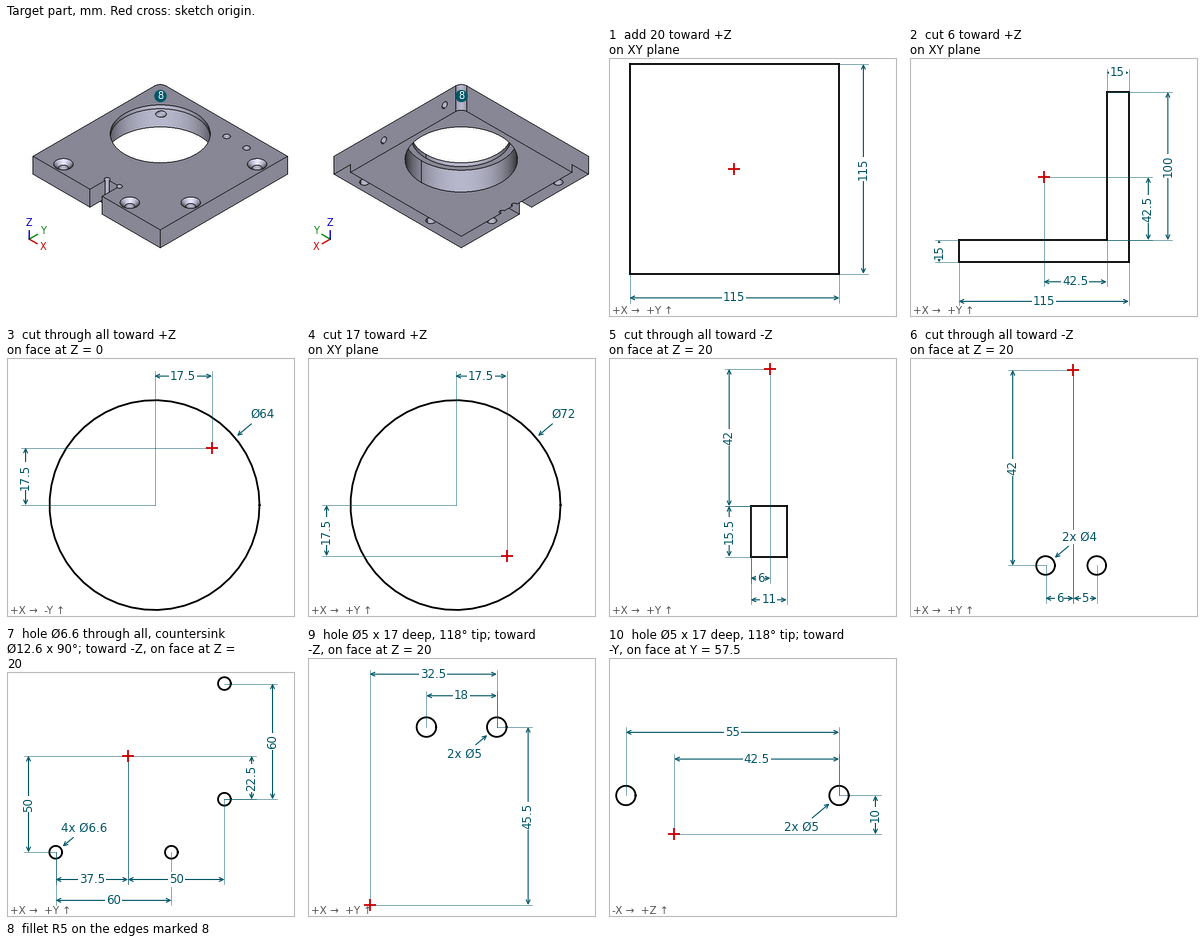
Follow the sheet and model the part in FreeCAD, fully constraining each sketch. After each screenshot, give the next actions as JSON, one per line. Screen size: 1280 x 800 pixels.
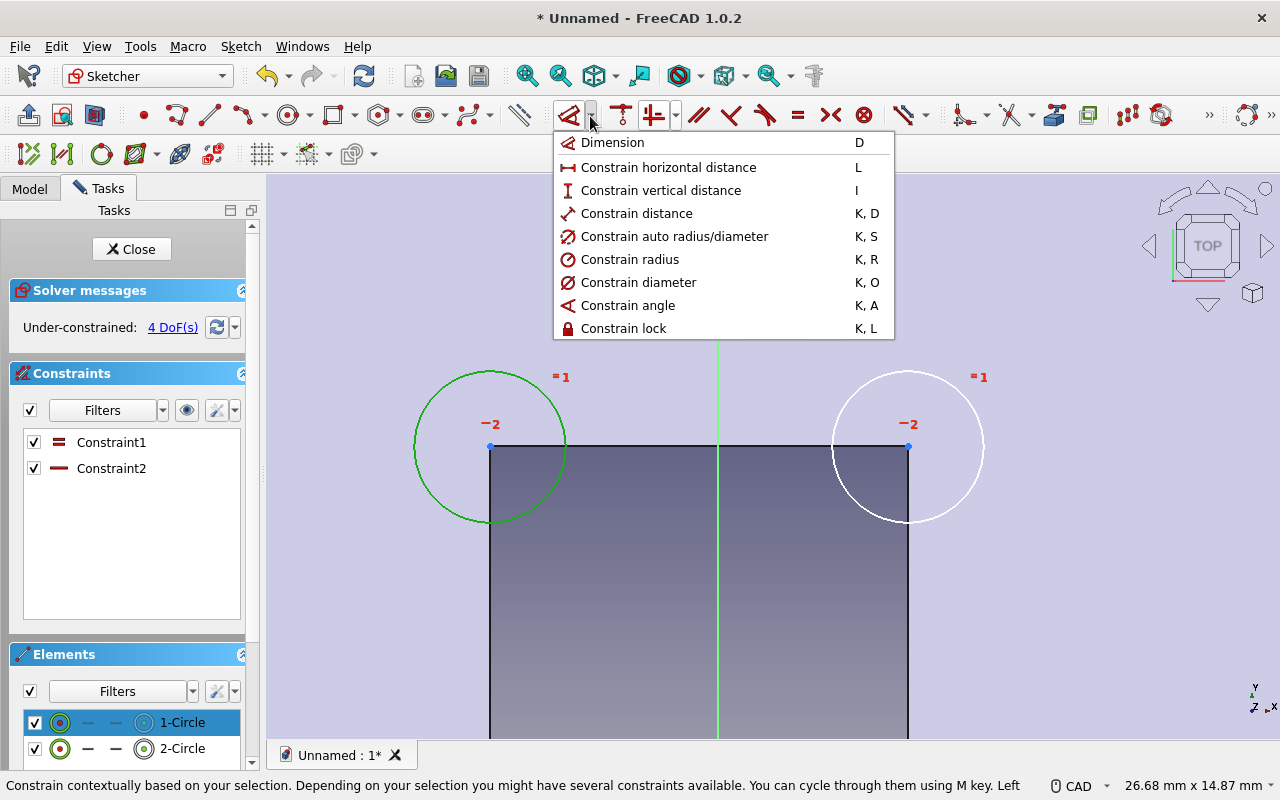
{"action": "left_click", "coordinate": [724, 282]}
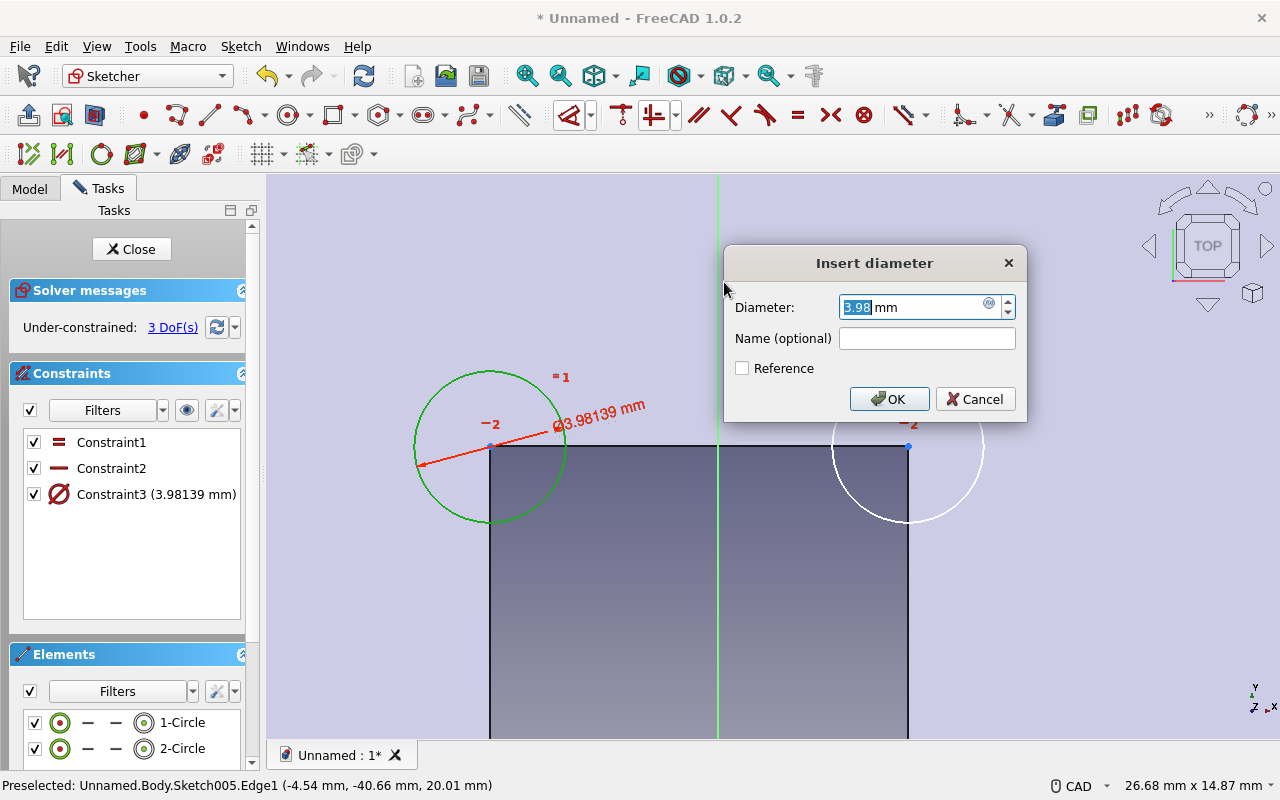
{"action": "type", "text": "4"}
{"action": "key", "text": "Return"}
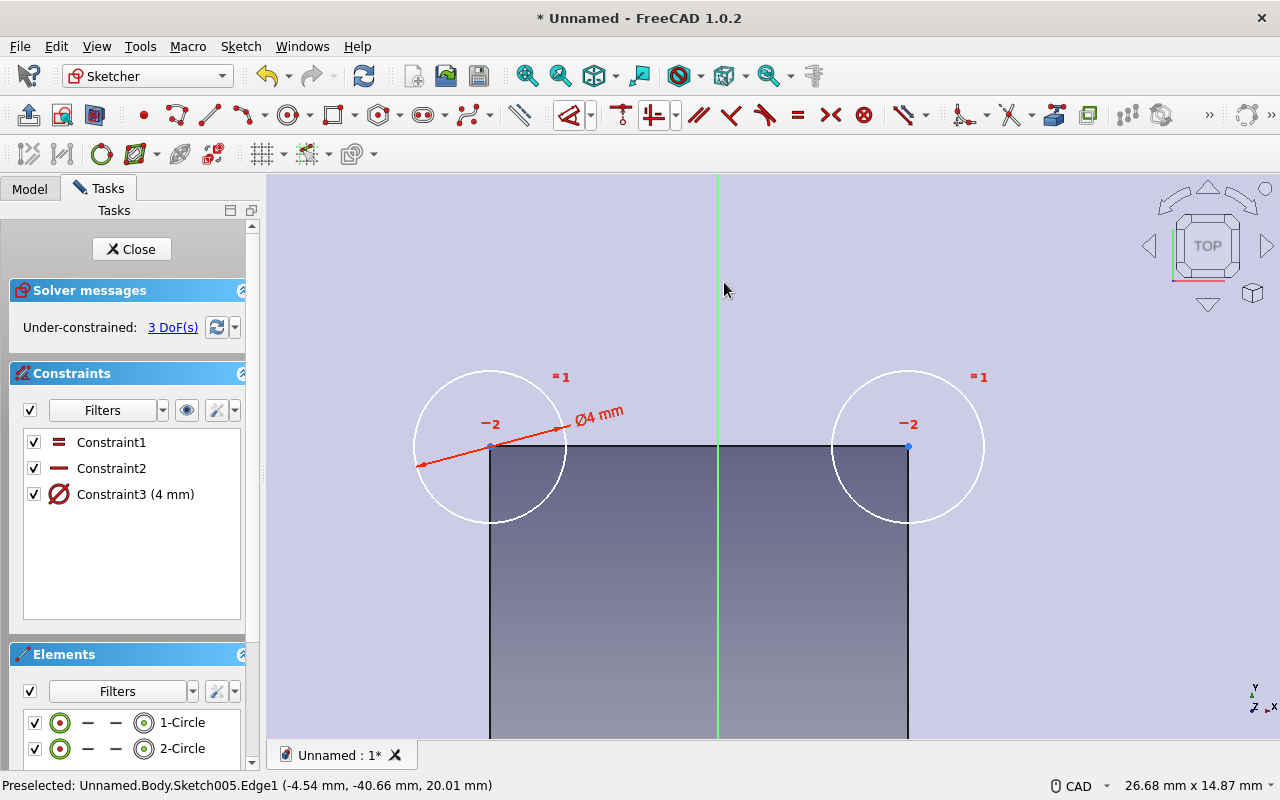
{"action": "left_click", "coordinate": [490, 447]}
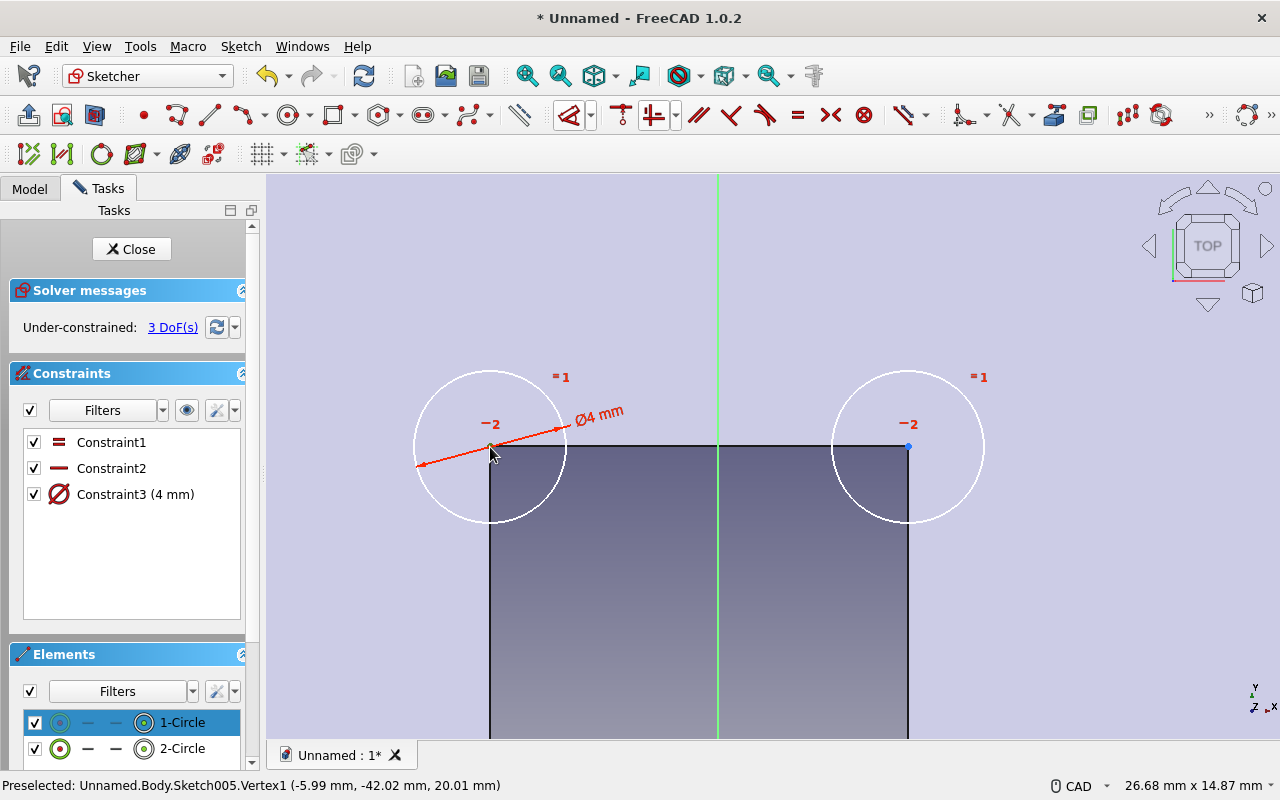
{"action": "key", "text": "l"}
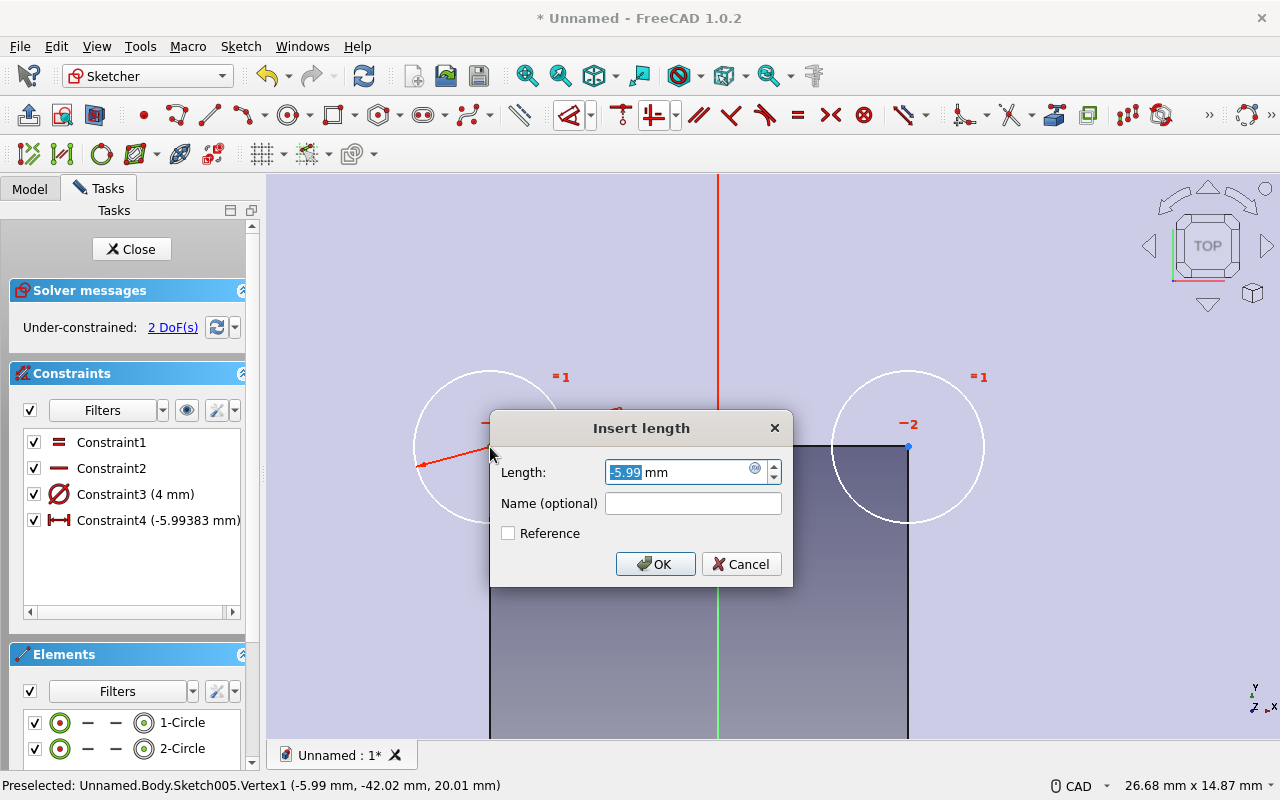
{"action": "type", "text": "-6"}
{"action": "key", "text": "Return"}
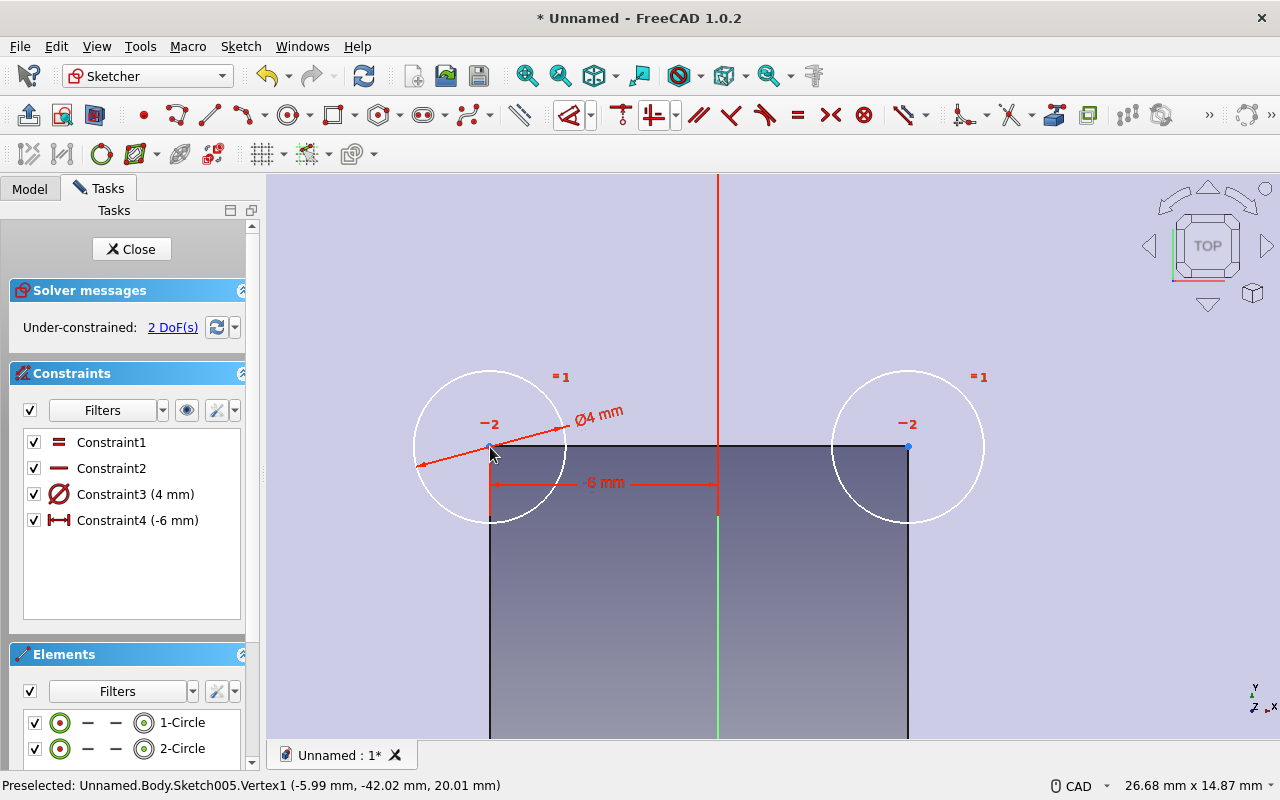
{"action": "left_click", "coordinate": [908, 447]}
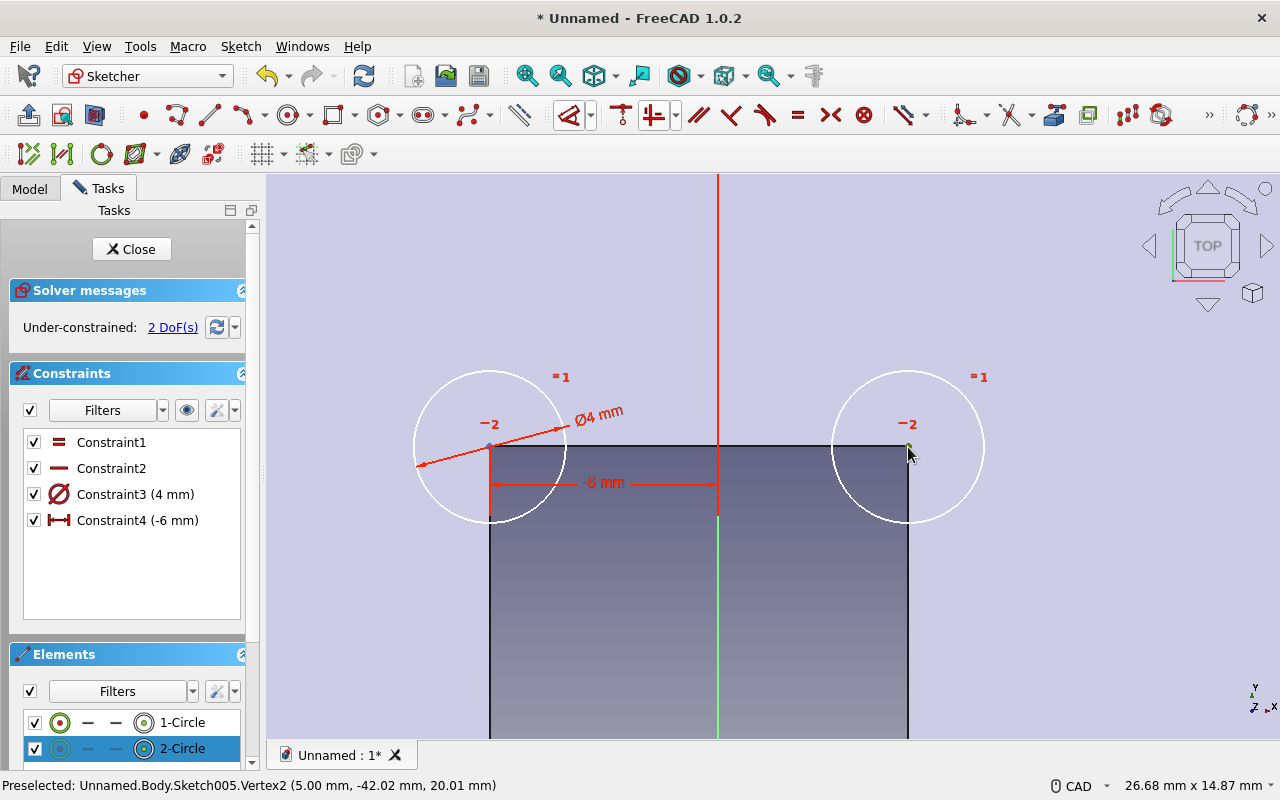
{"action": "key", "text": "l"}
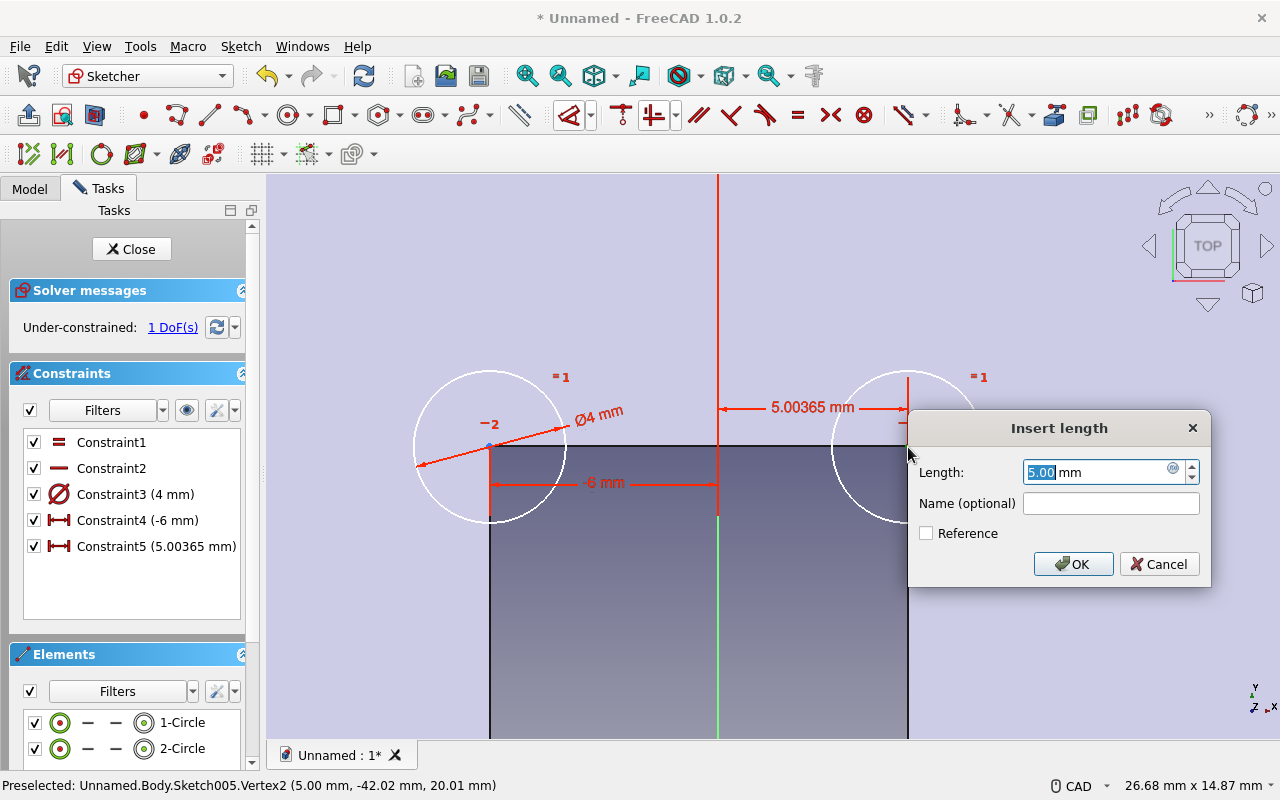
{"action": "type", "text": "5"}
{"action": "key", "text": "Return"}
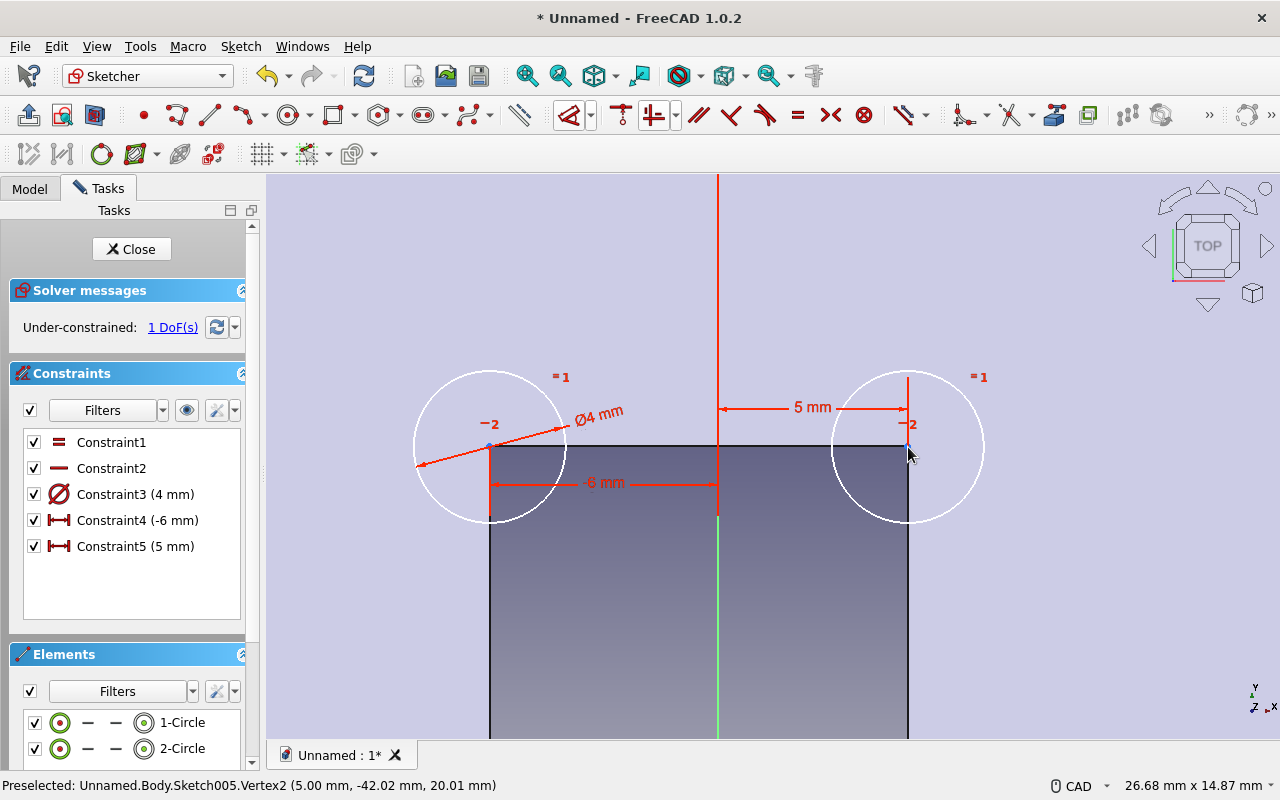
{"action": "left_click", "coordinate": [490, 447]}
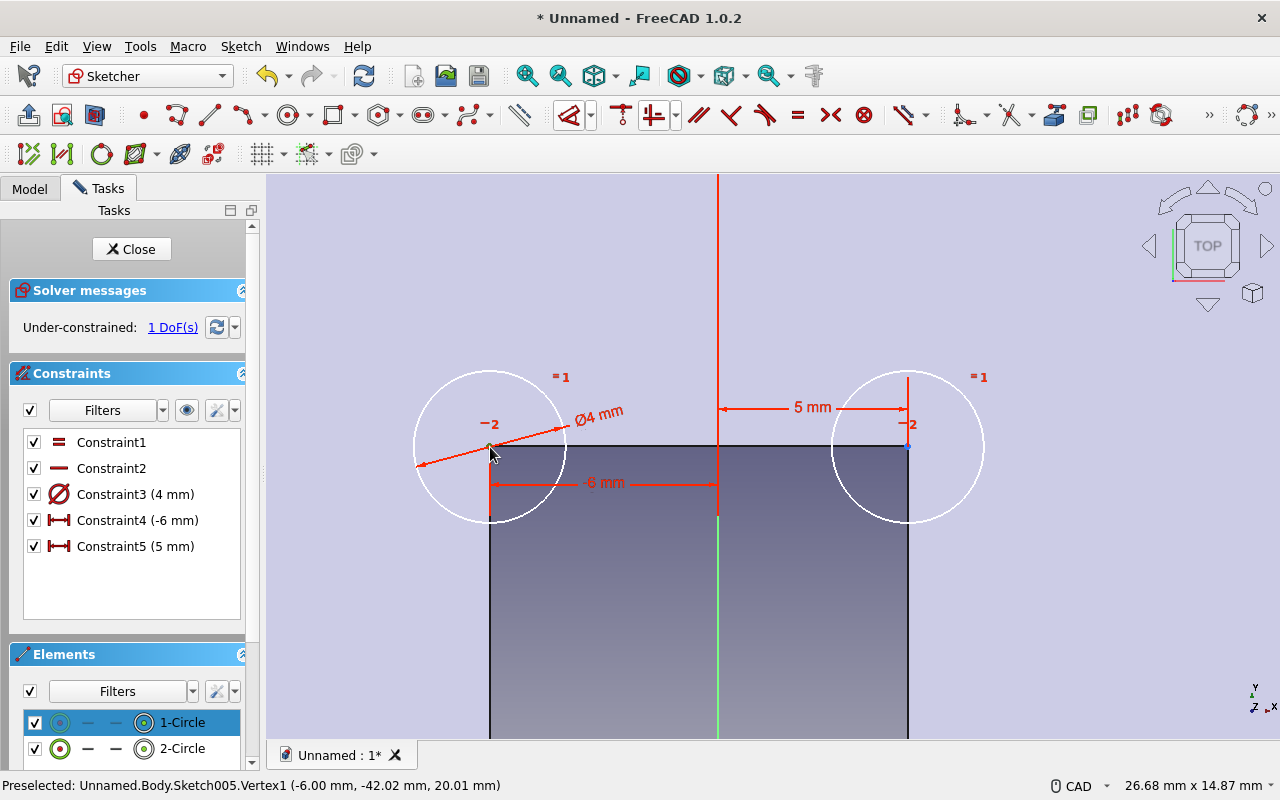
{"action": "key", "text": "i"}